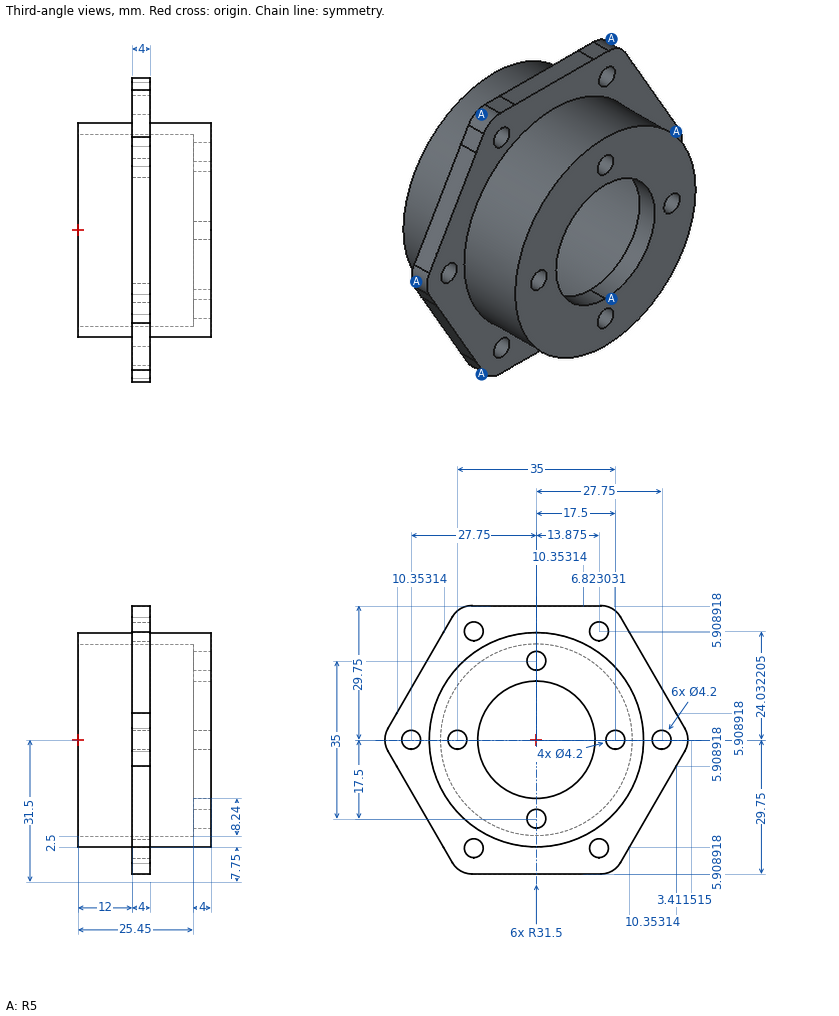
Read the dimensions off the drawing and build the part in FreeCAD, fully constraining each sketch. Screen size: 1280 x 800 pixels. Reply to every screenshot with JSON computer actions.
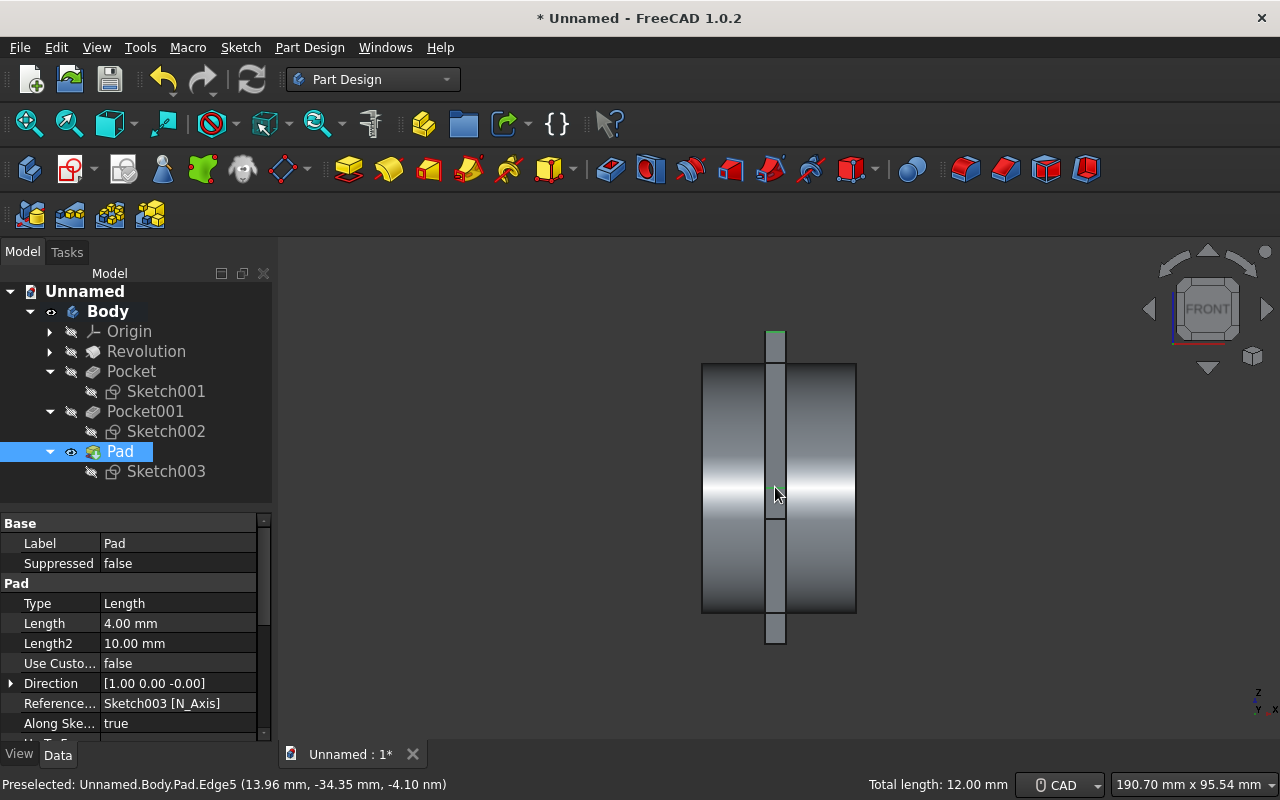
{"action": "scroll", "coordinate": [775, 643], "scroll_direction": "up", "scroll_amount": 4}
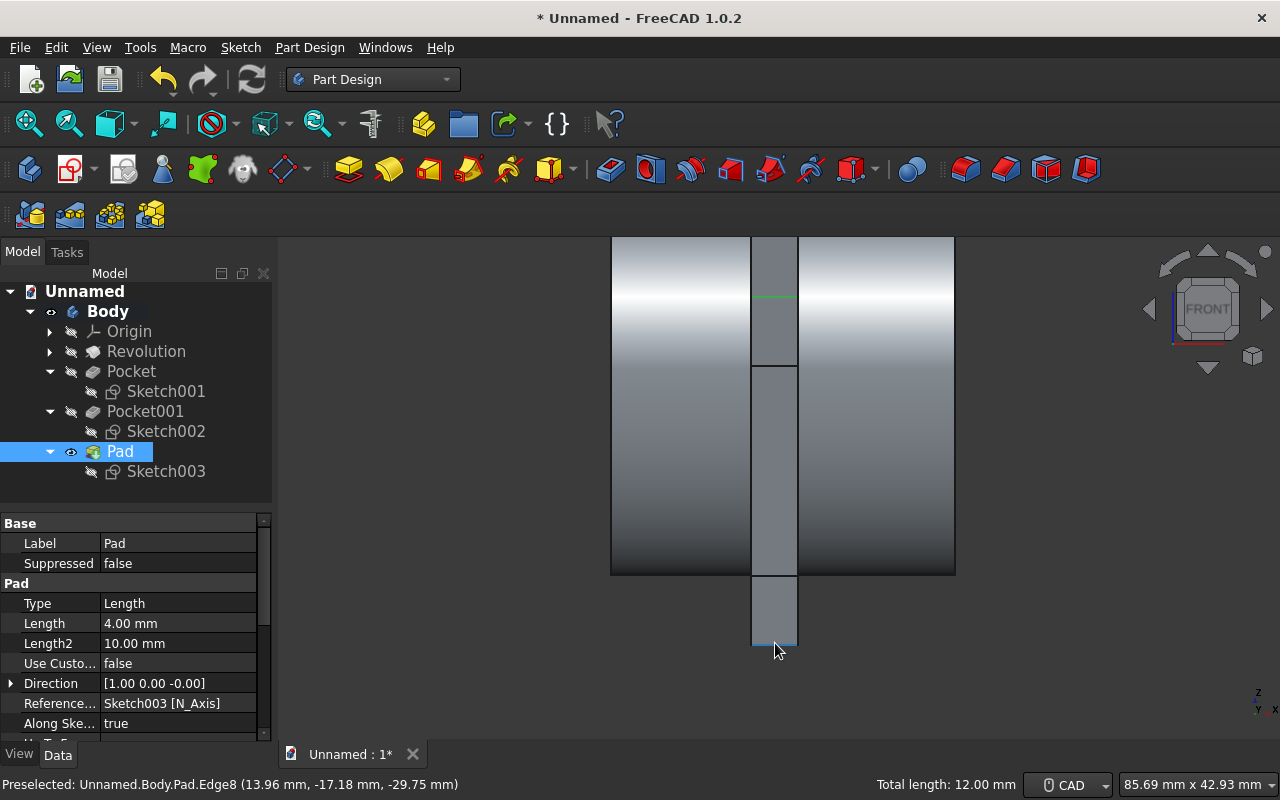
{"action": "key", "text": "v f"}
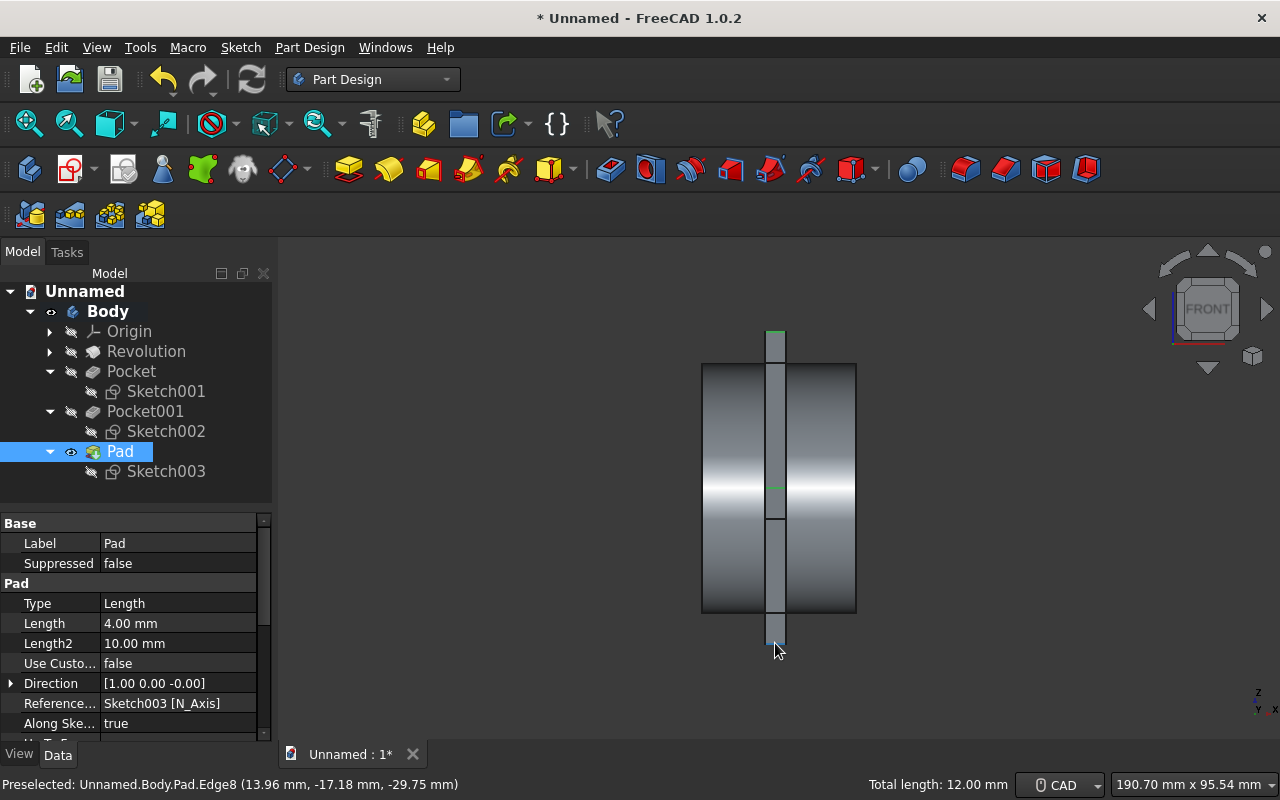
{"action": "key", "text": "3"}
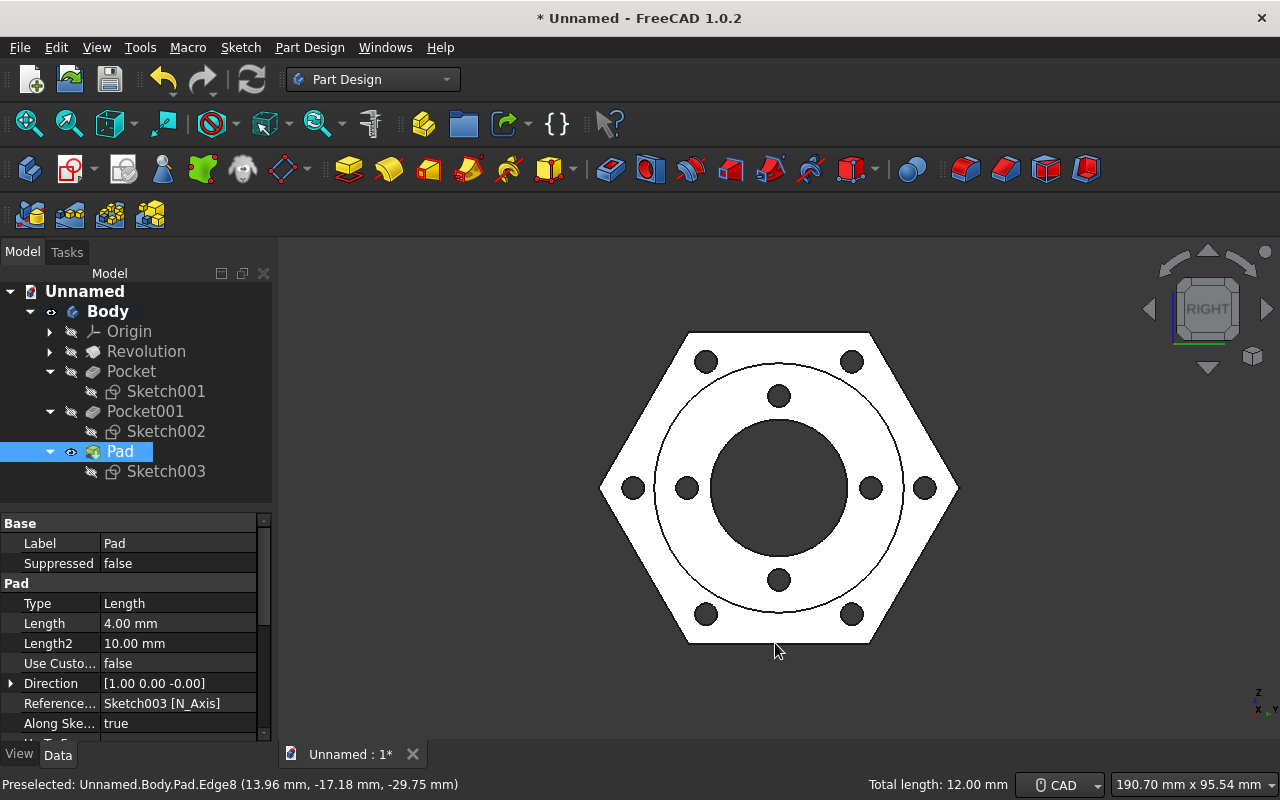
{"action": "scroll", "coordinate": [689, 643], "scroll_direction": "up", "scroll_amount": 4}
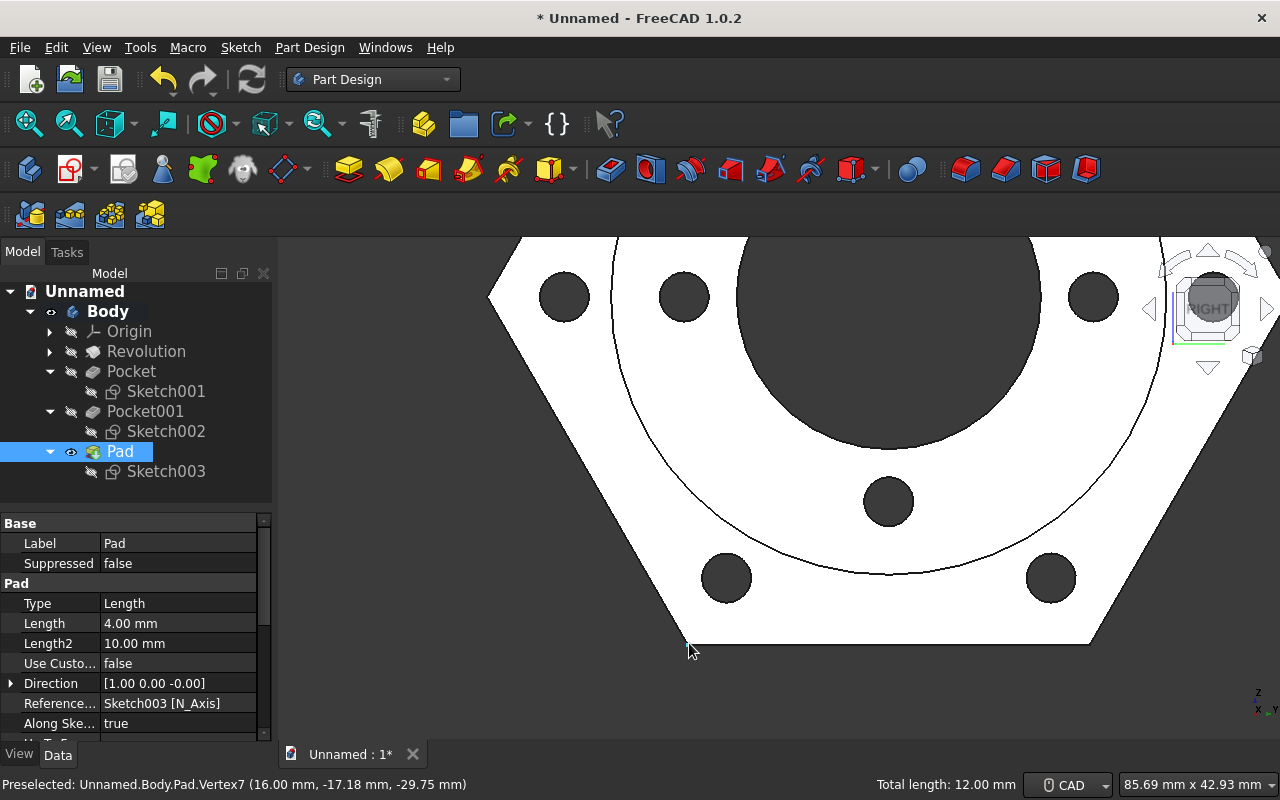
{"action": "key", "text": "v f"}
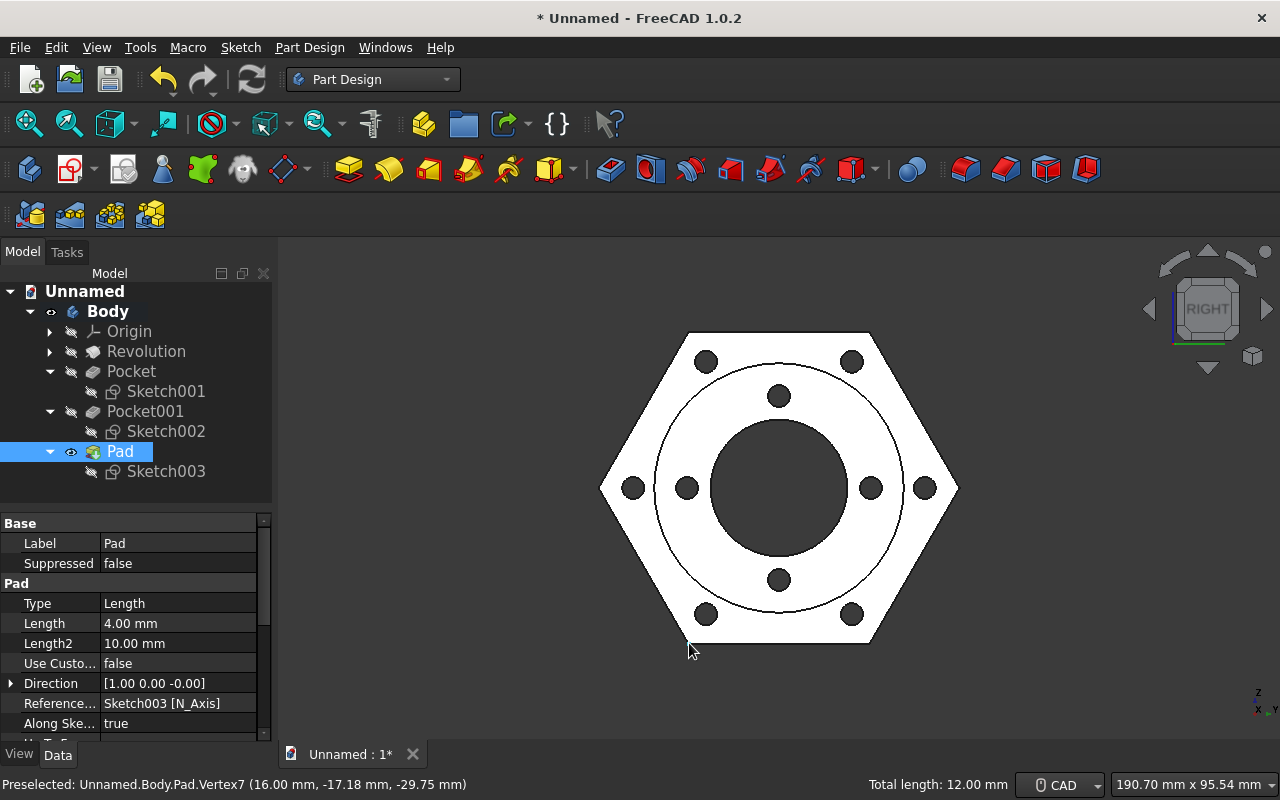
{"action": "key", "text": "5"}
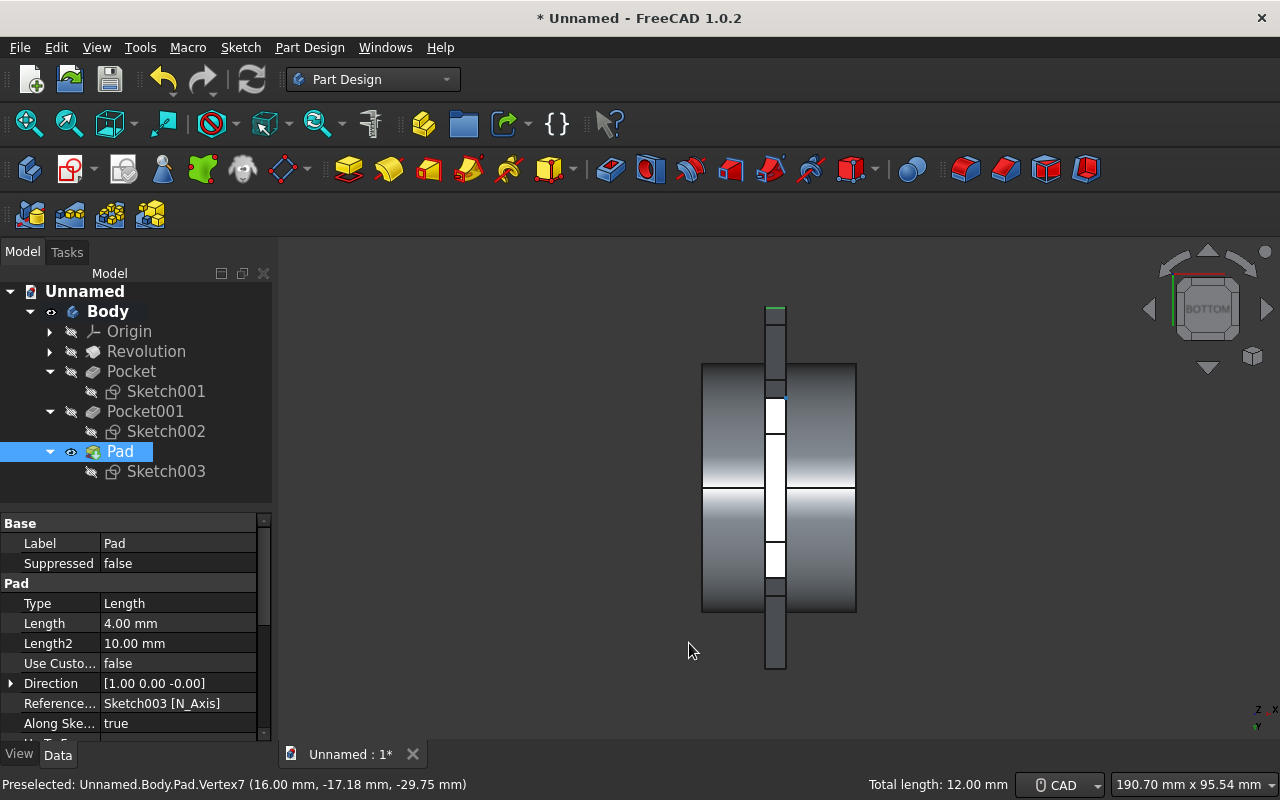
{"action": "left_click", "coordinate": [775, 397], "text": "ctrl"}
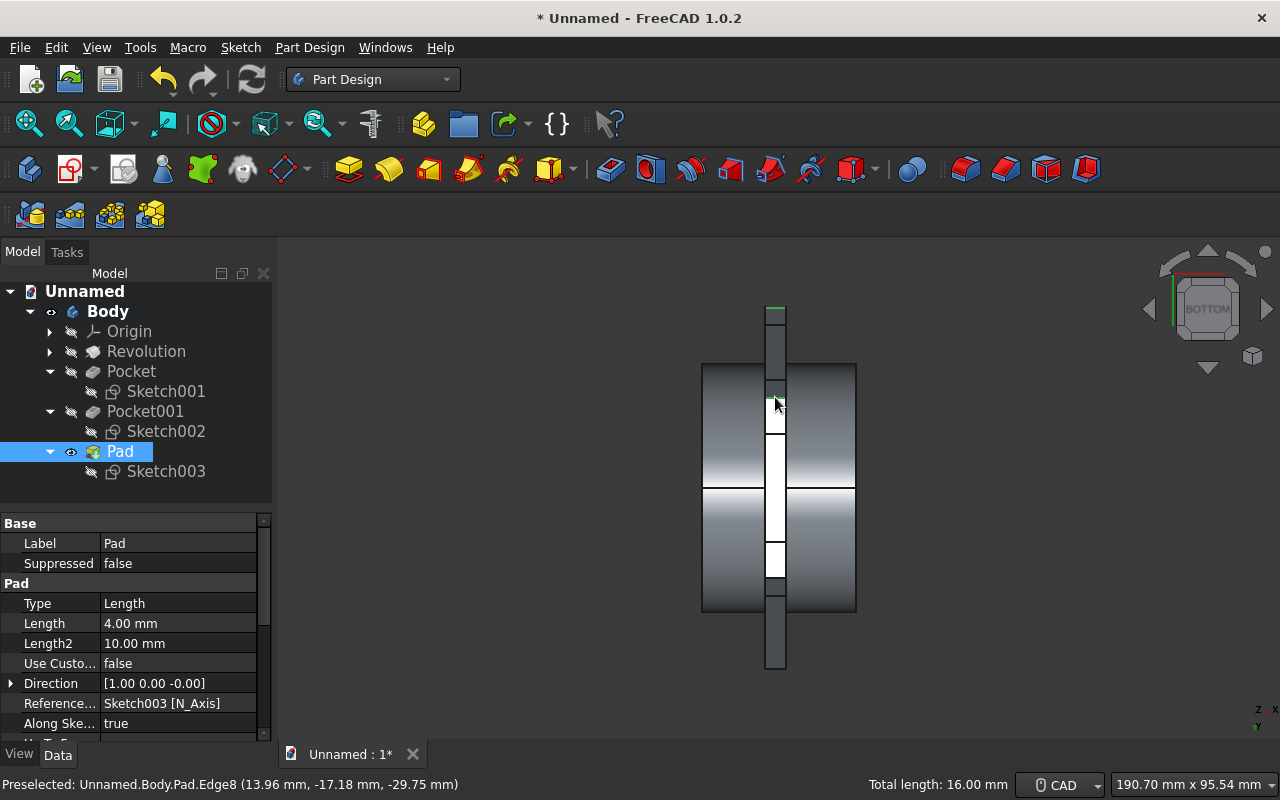
{"action": "scroll", "coordinate": [775, 577], "scroll_direction": "up", "scroll_amount": 4}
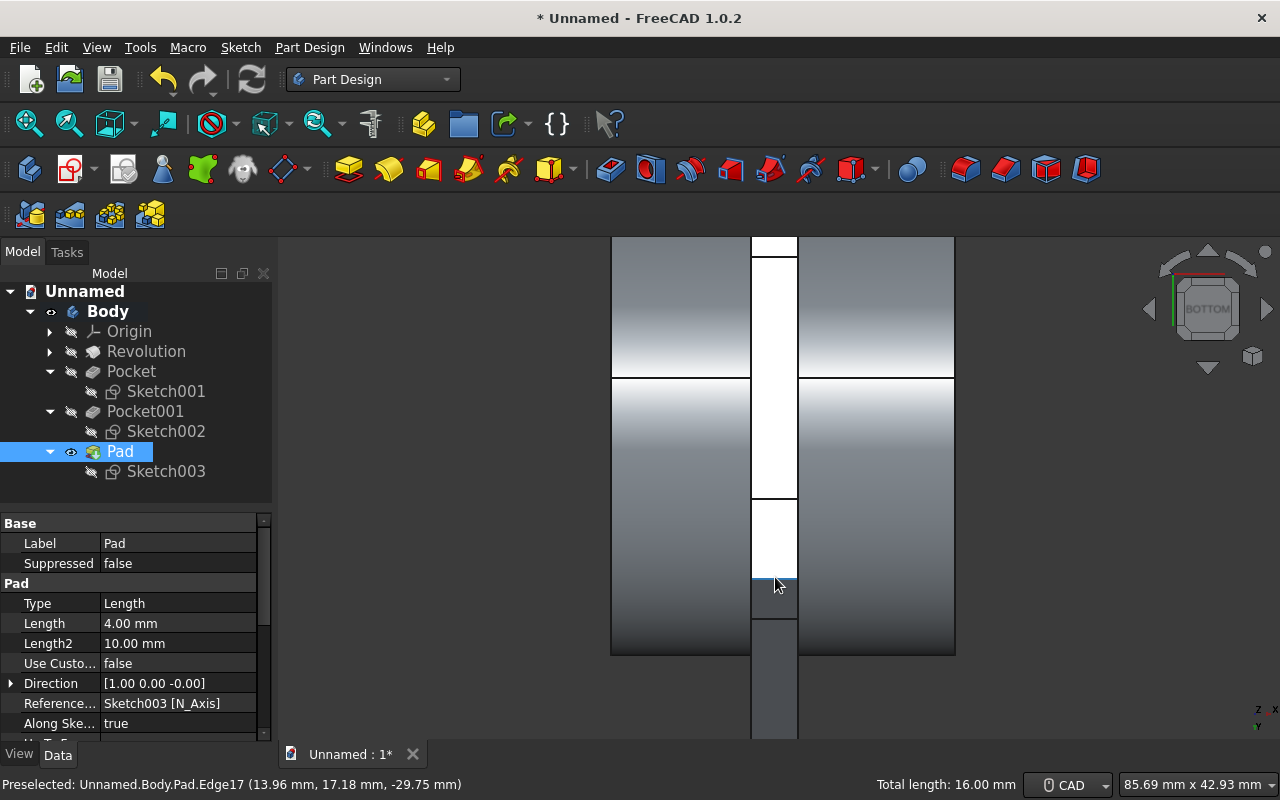
{"action": "left_click", "coordinate": [30, 124]}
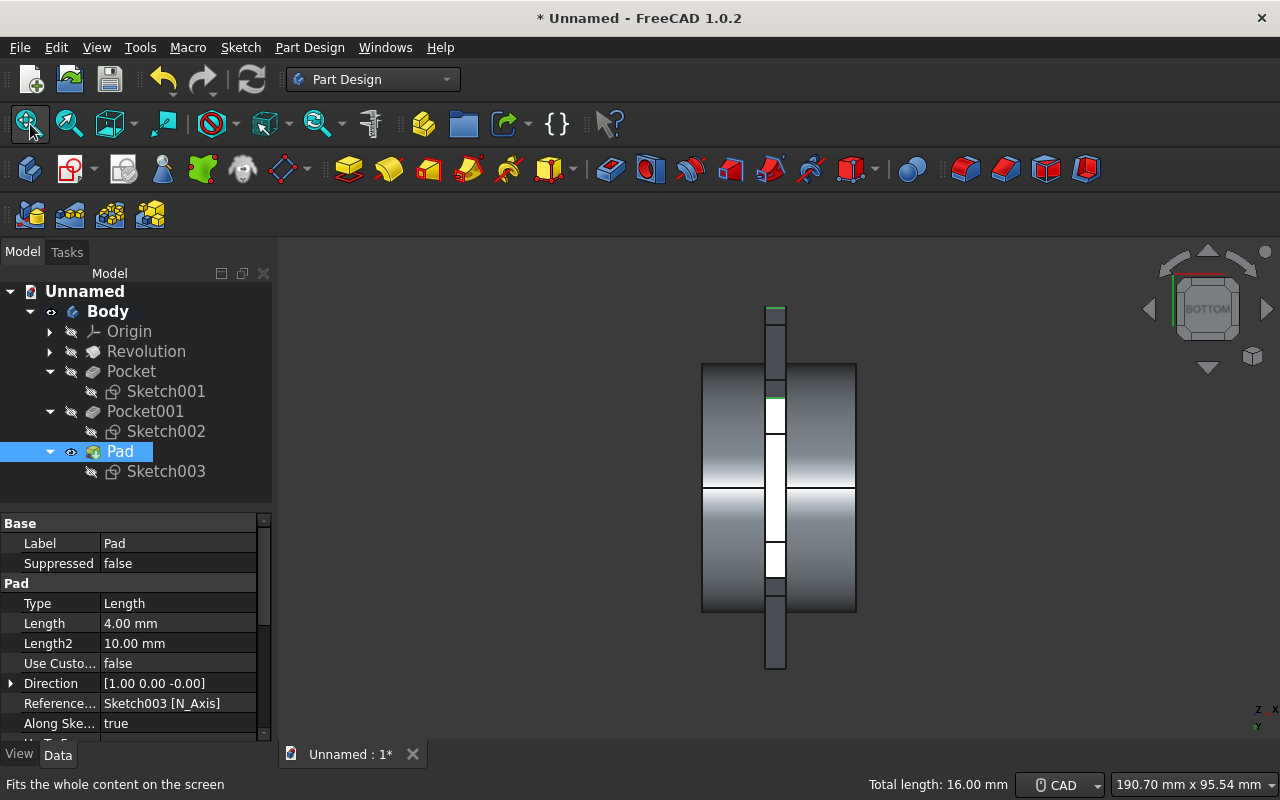
{"action": "key", "text": "4"}